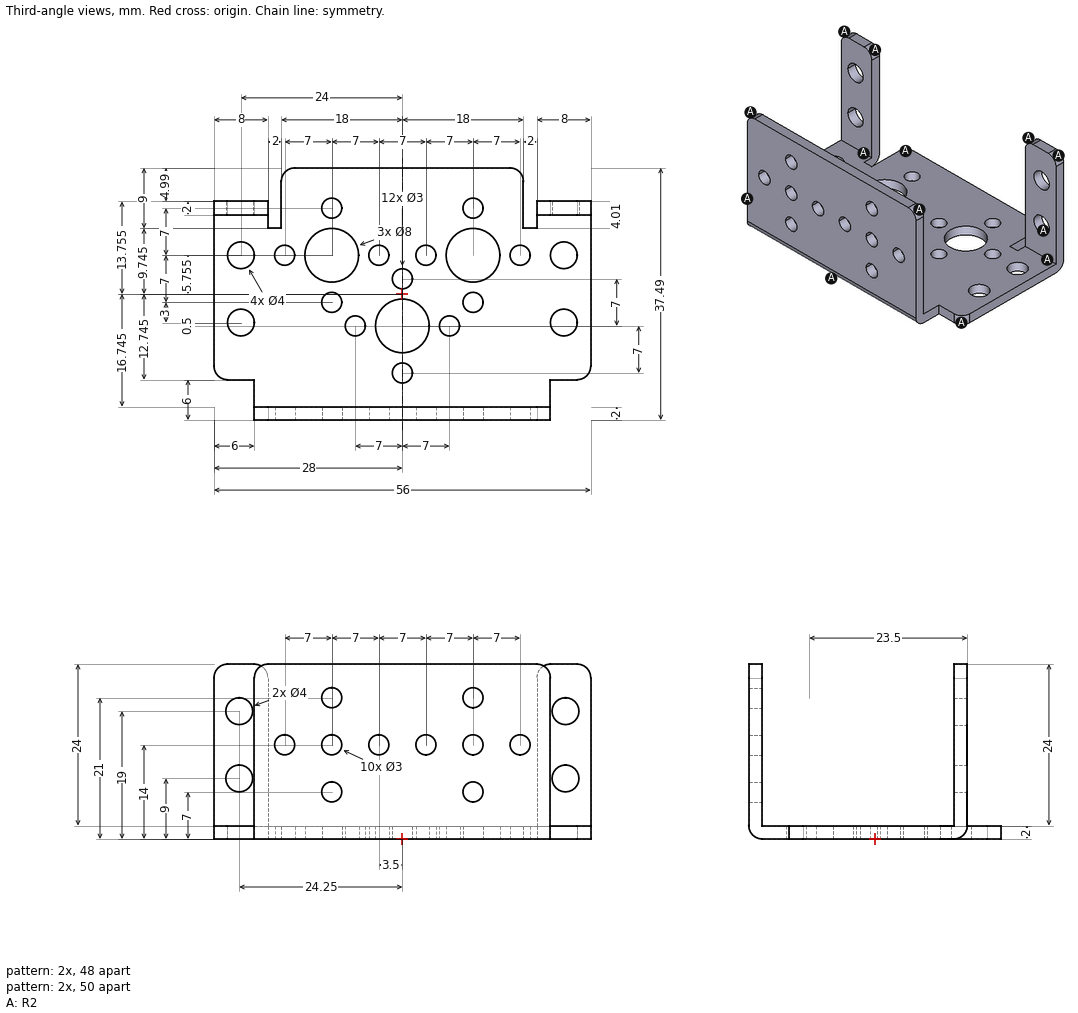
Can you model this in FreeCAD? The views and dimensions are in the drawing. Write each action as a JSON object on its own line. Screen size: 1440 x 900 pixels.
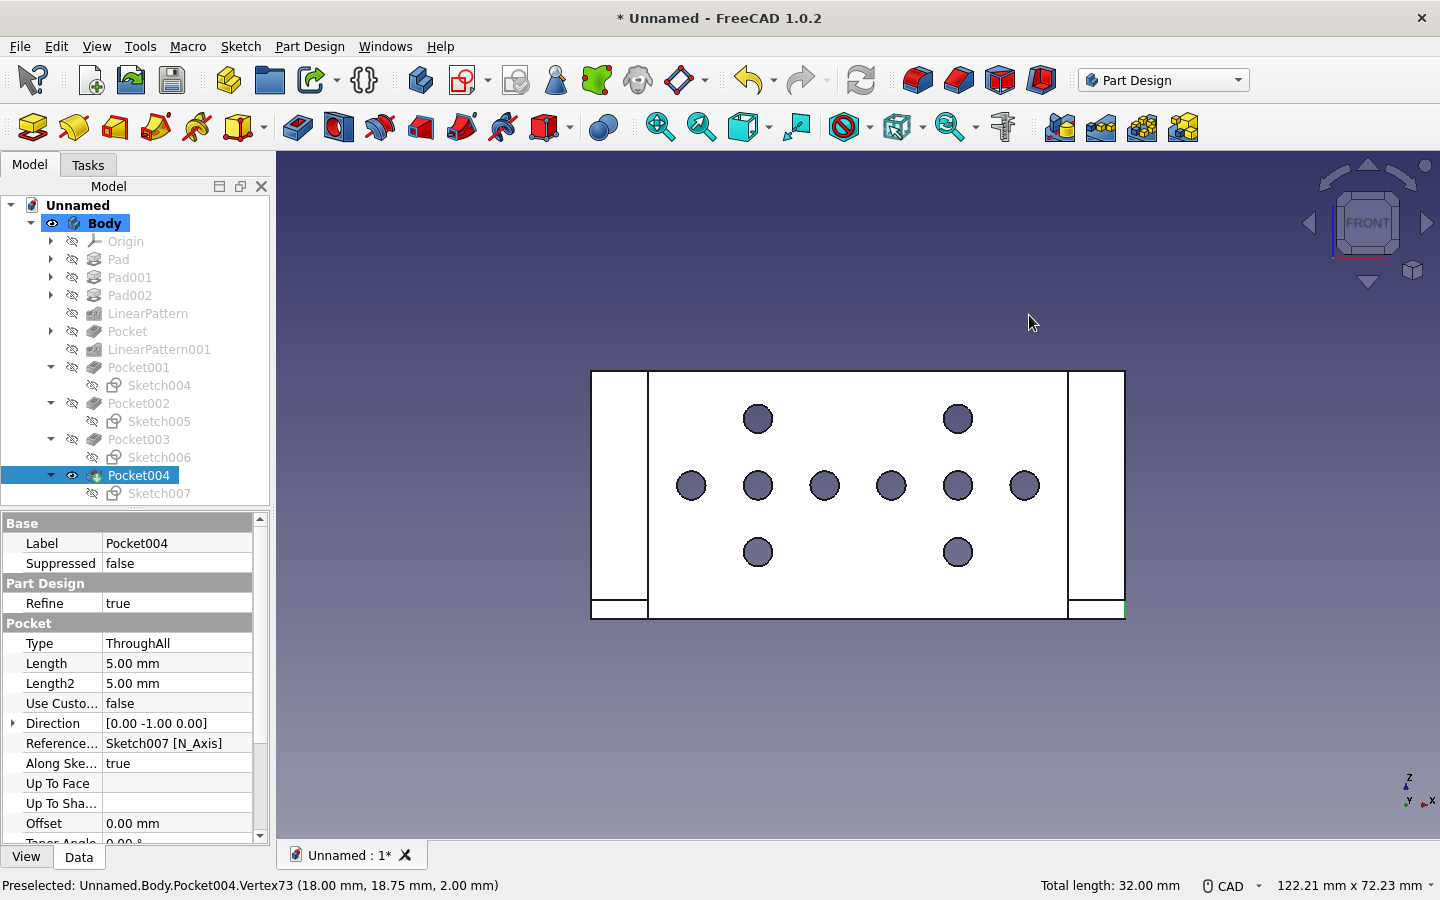
{"action": "left_click", "coordinate": [858, 618], "text": "ctrl"}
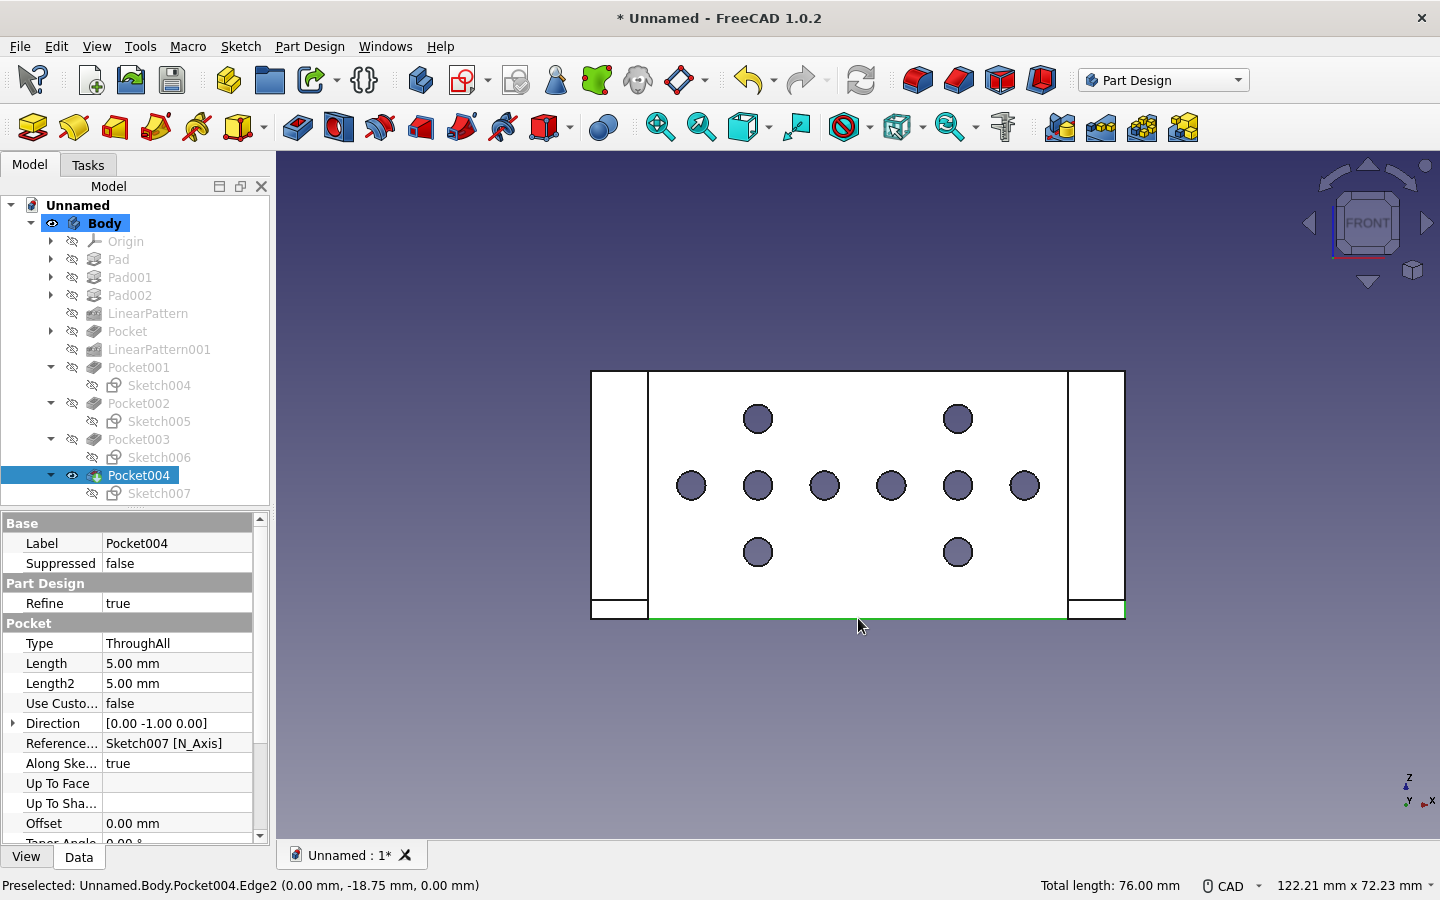
{"action": "left_click", "coordinate": [591, 608], "text": "ctrl"}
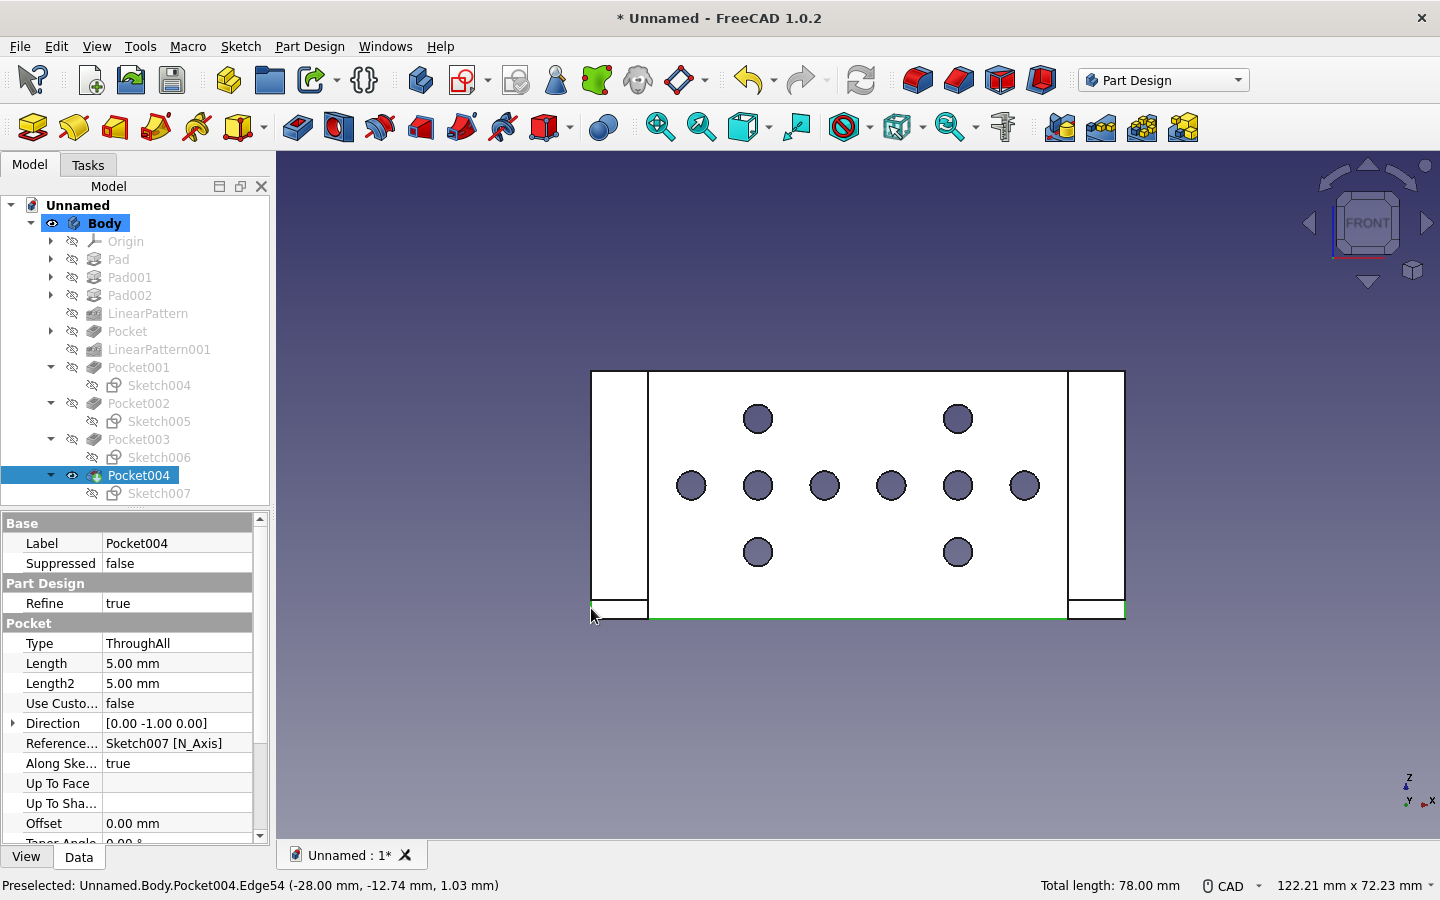
{"action": "scroll", "coordinate": [1029, 608], "scroll_direction": "up", "scroll_amount": 4}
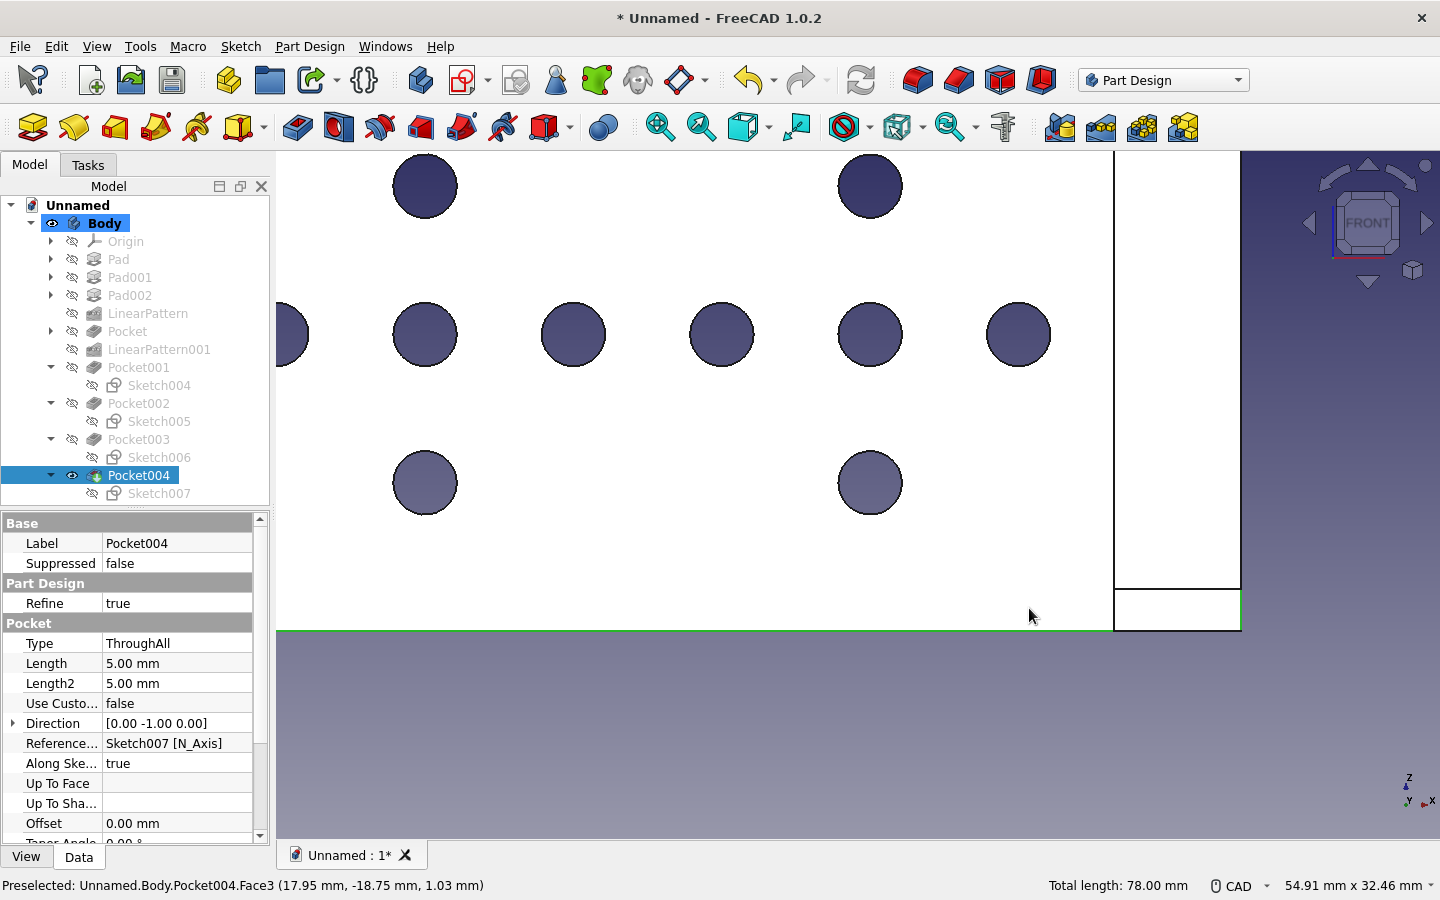
{"action": "key", "text": "v f"}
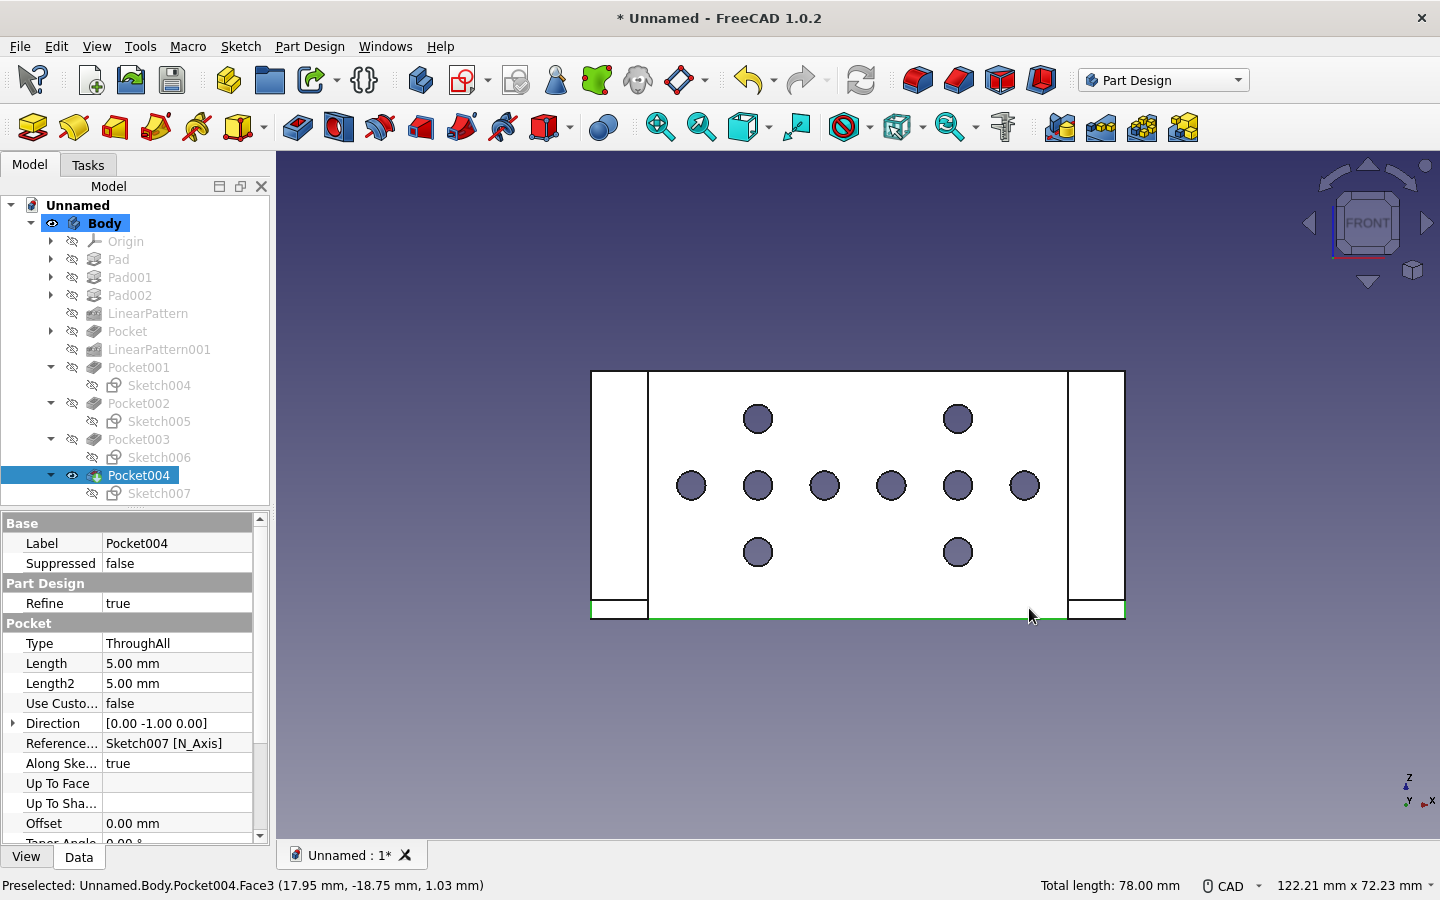
{"action": "key", "text": "3"}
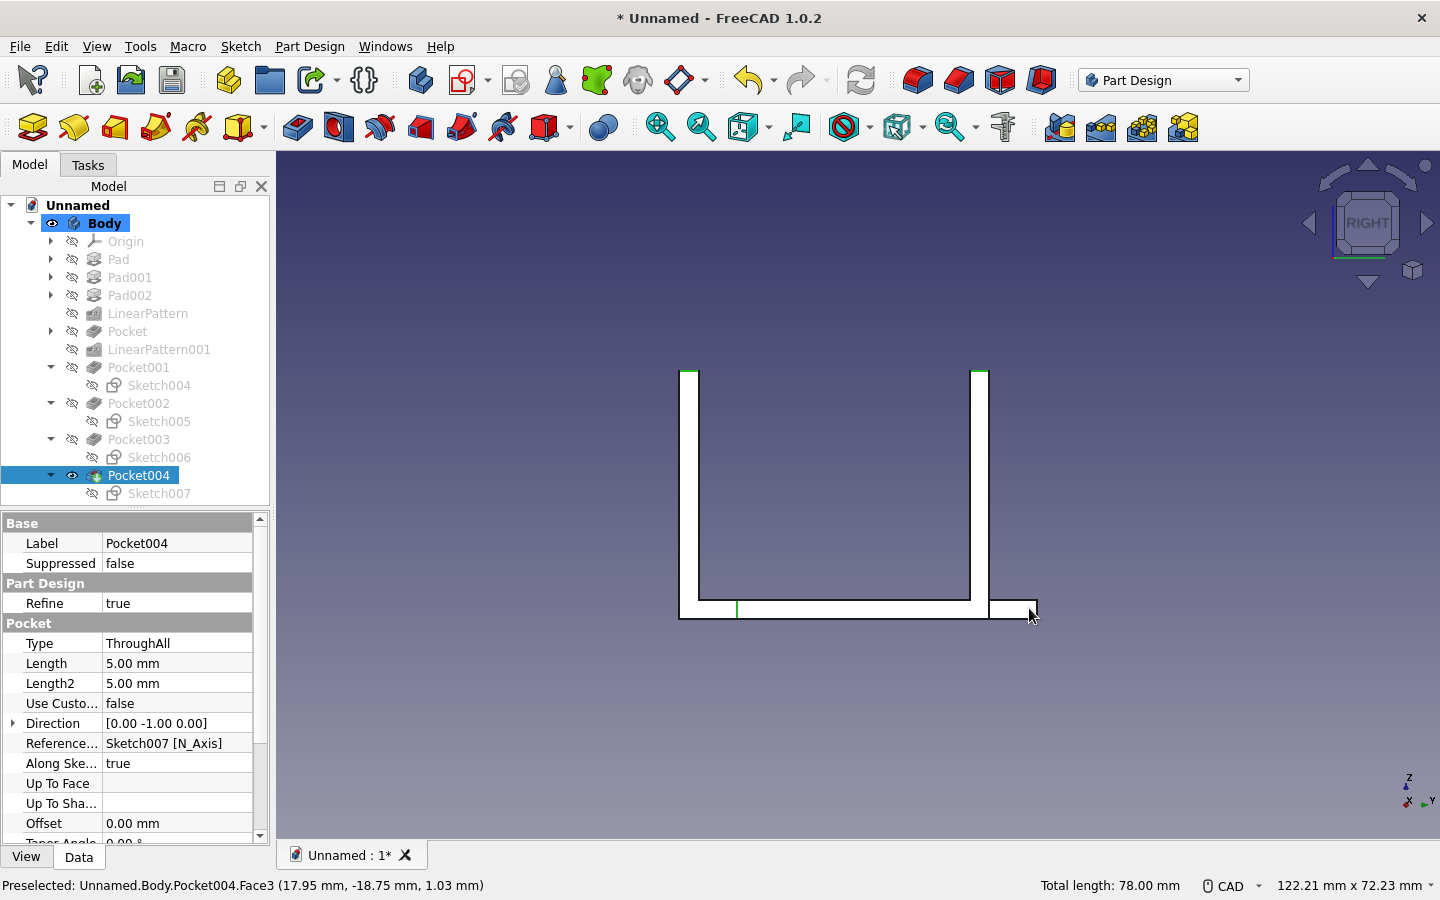
{"action": "key", "text": "v f"}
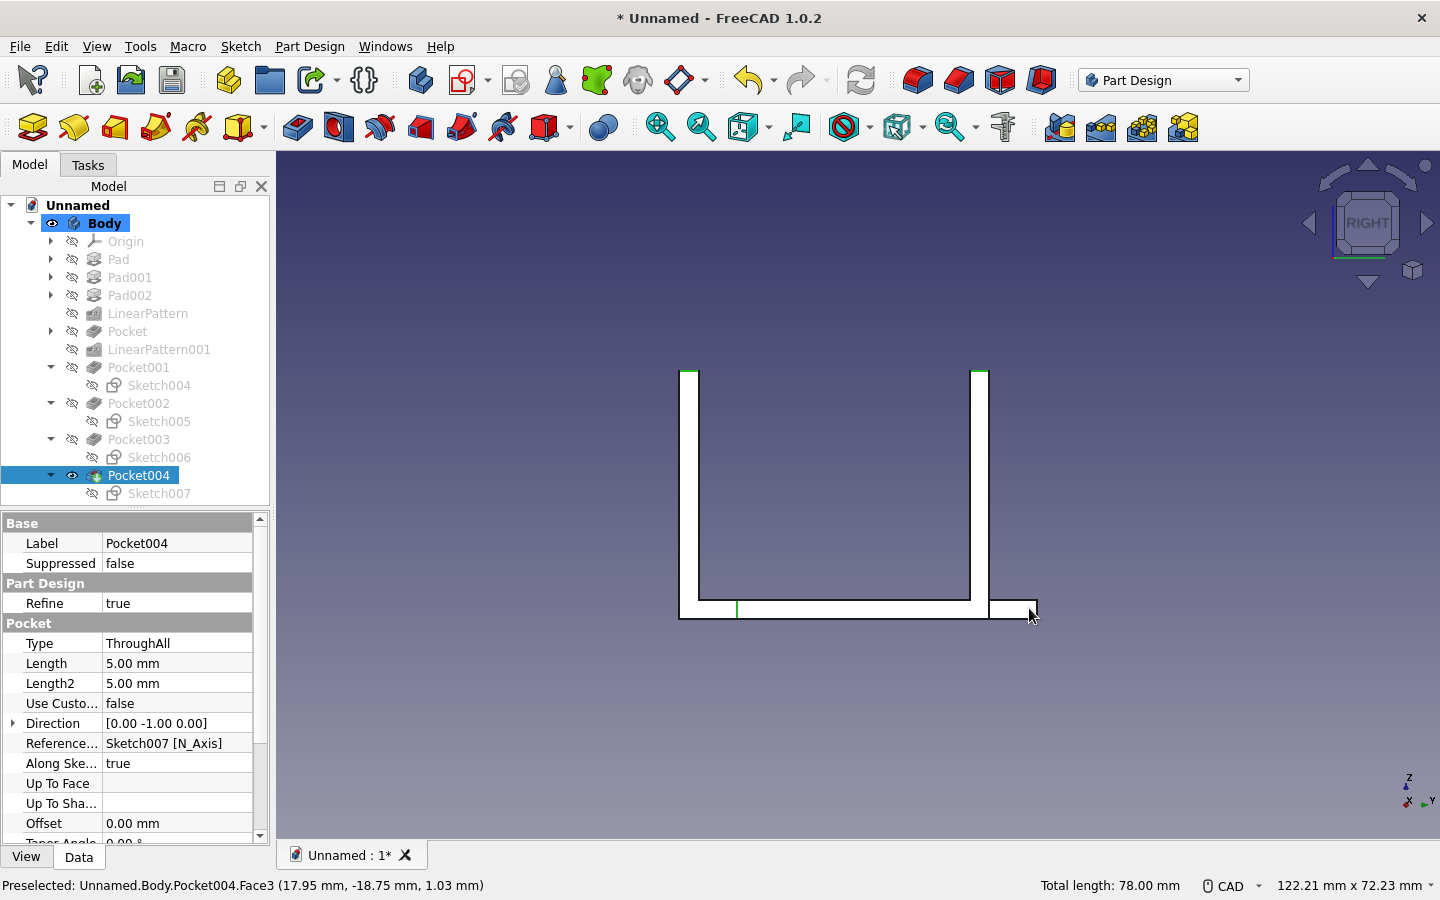
{"action": "left_click", "coordinate": [1037, 608], "text": "ctrl"}